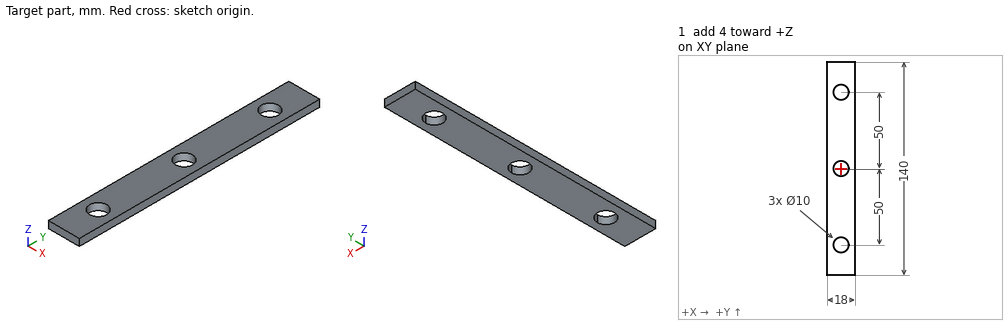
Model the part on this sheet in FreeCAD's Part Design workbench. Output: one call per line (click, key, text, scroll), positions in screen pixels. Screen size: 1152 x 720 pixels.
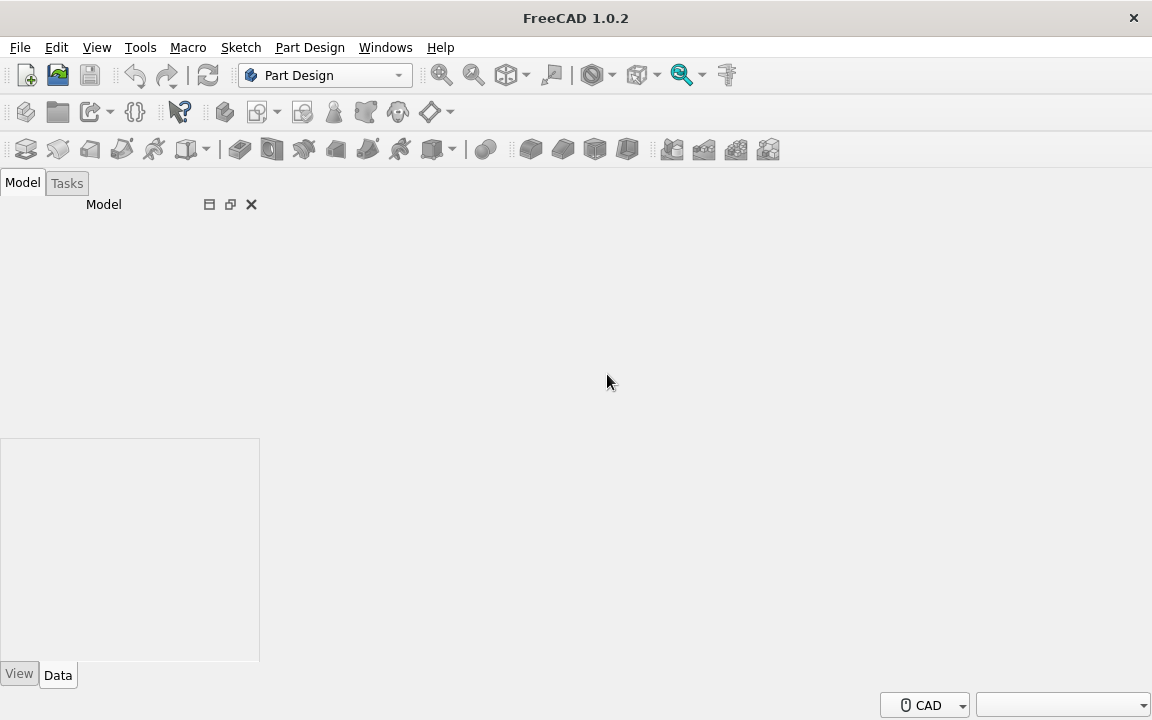
key(ctrl+n)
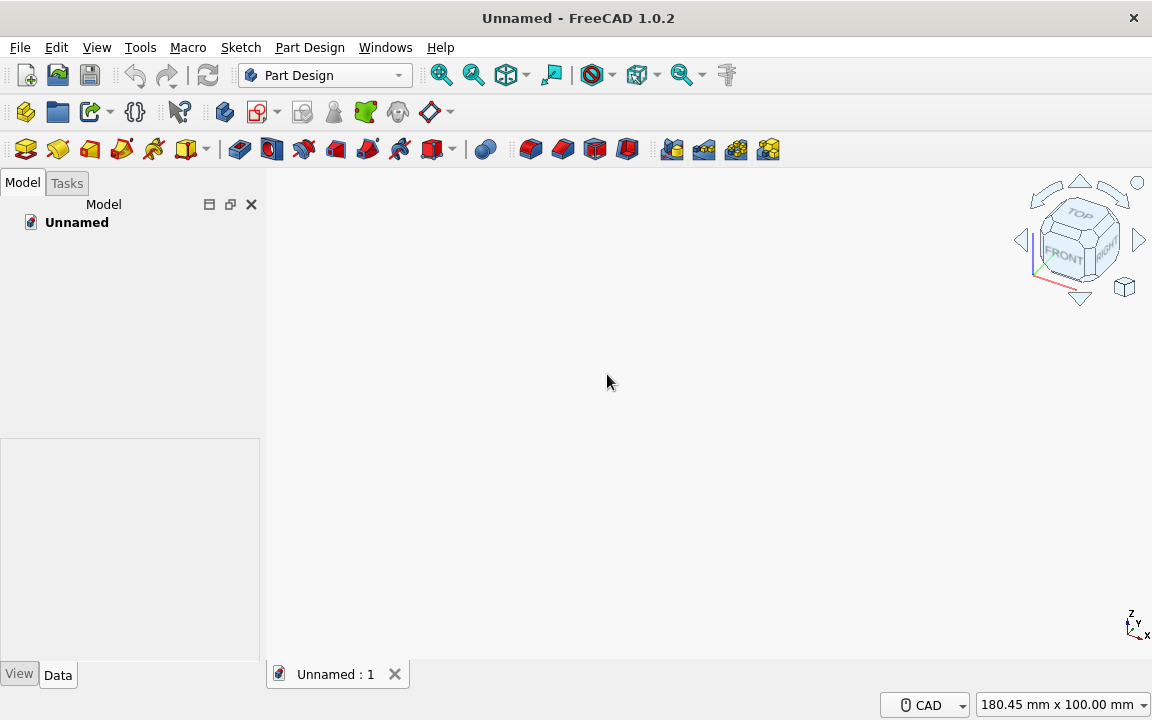
click(258, 112)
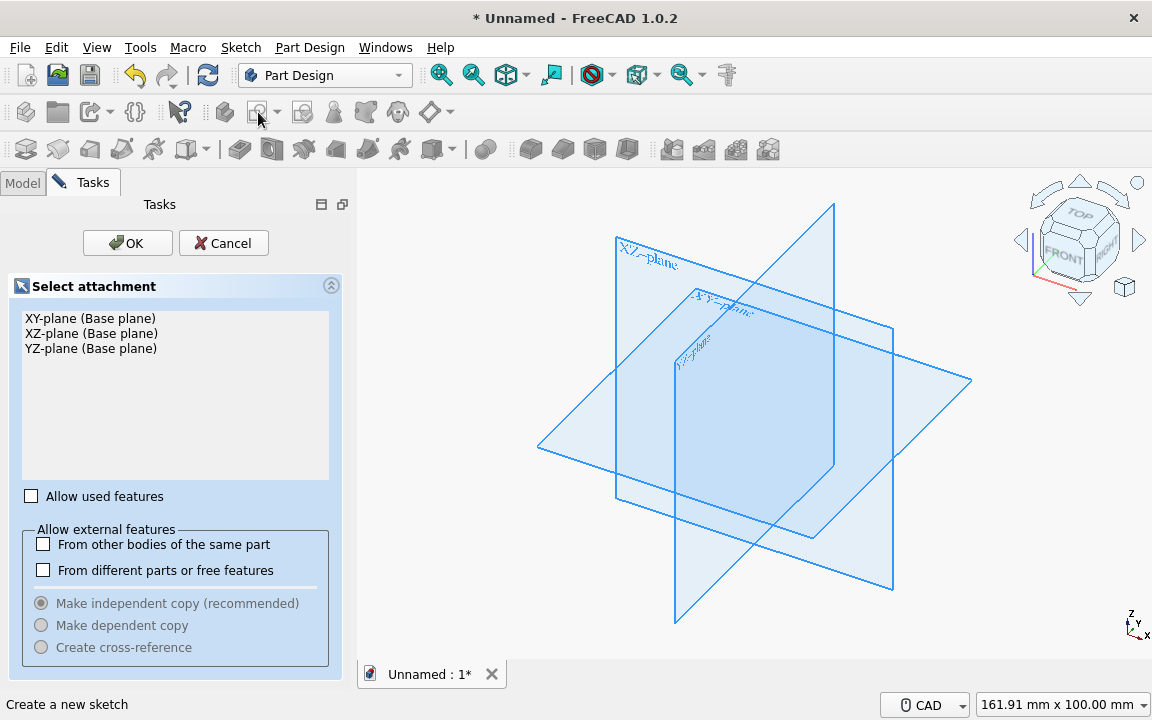
click(82, 318)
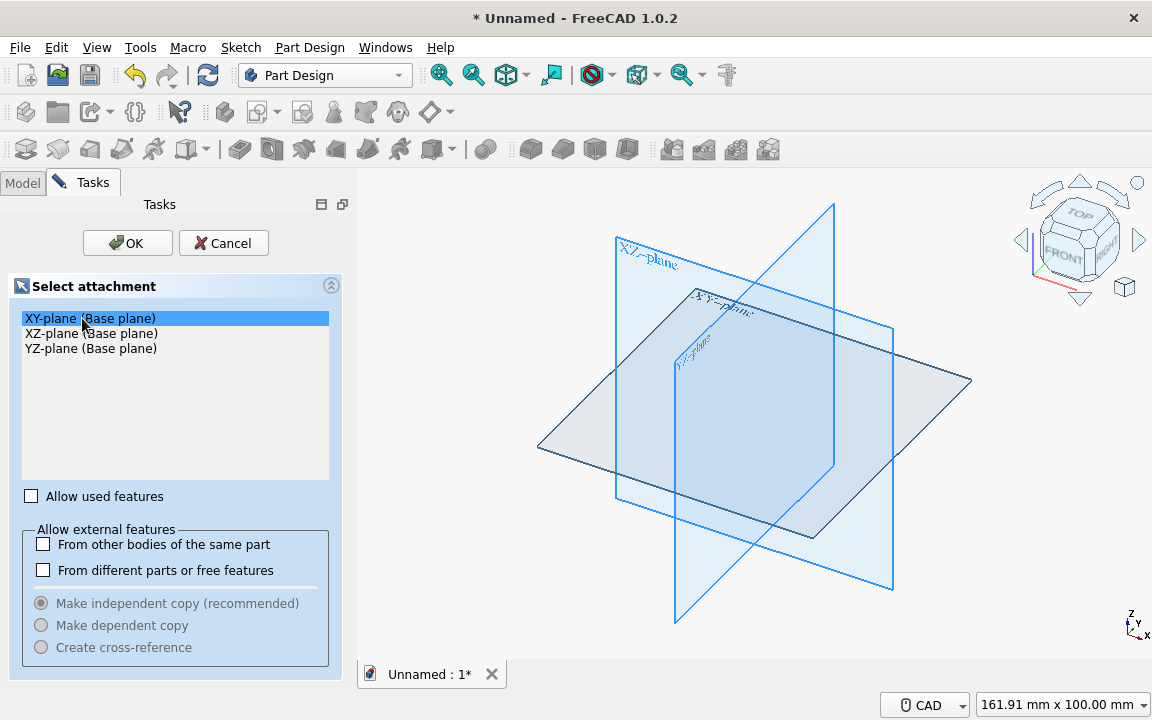
click(128, 243)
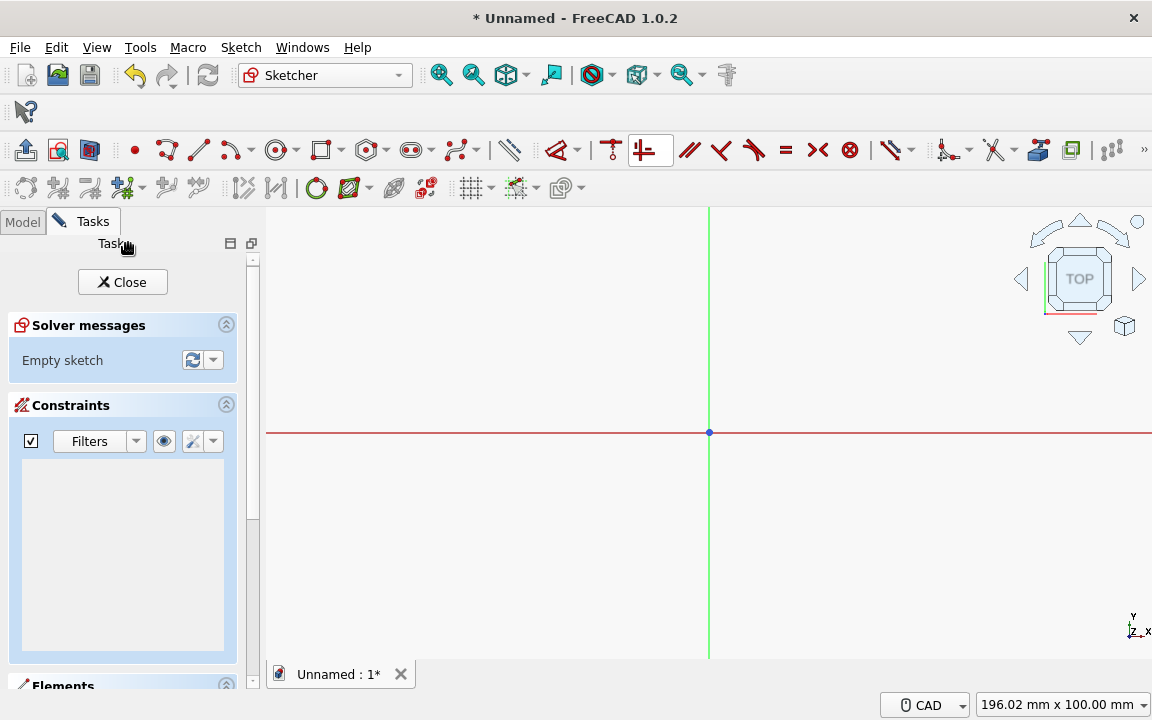
scroll(585, 433, down, 4)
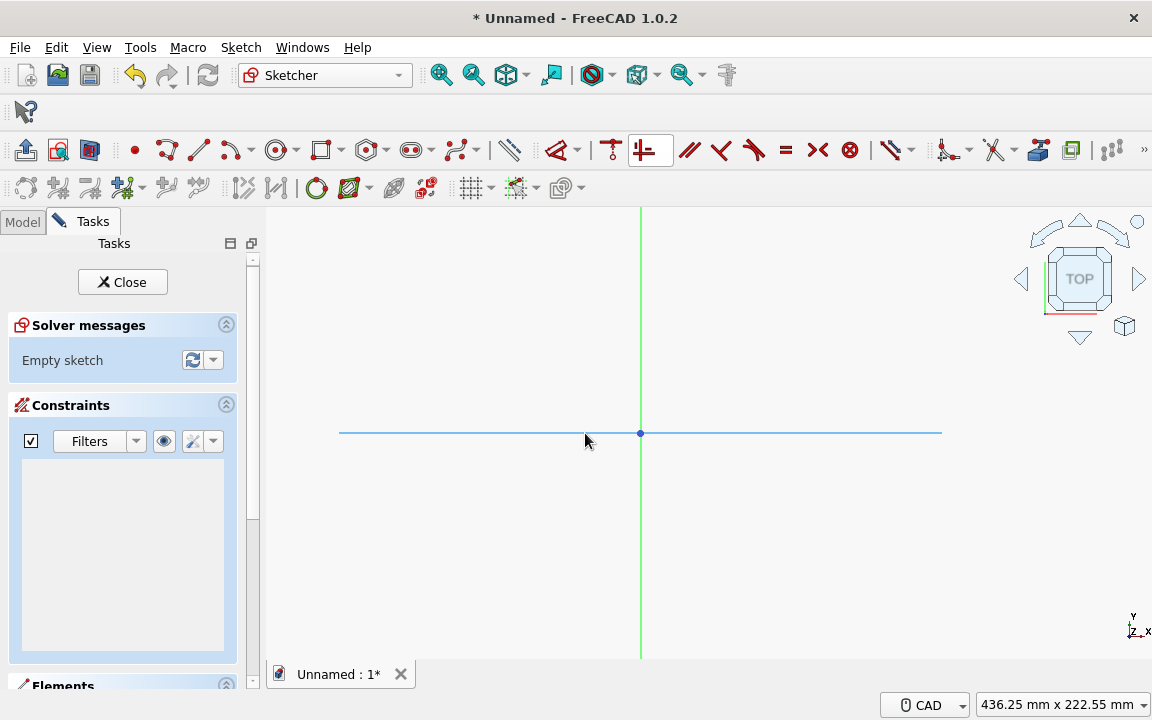
click(344, 150)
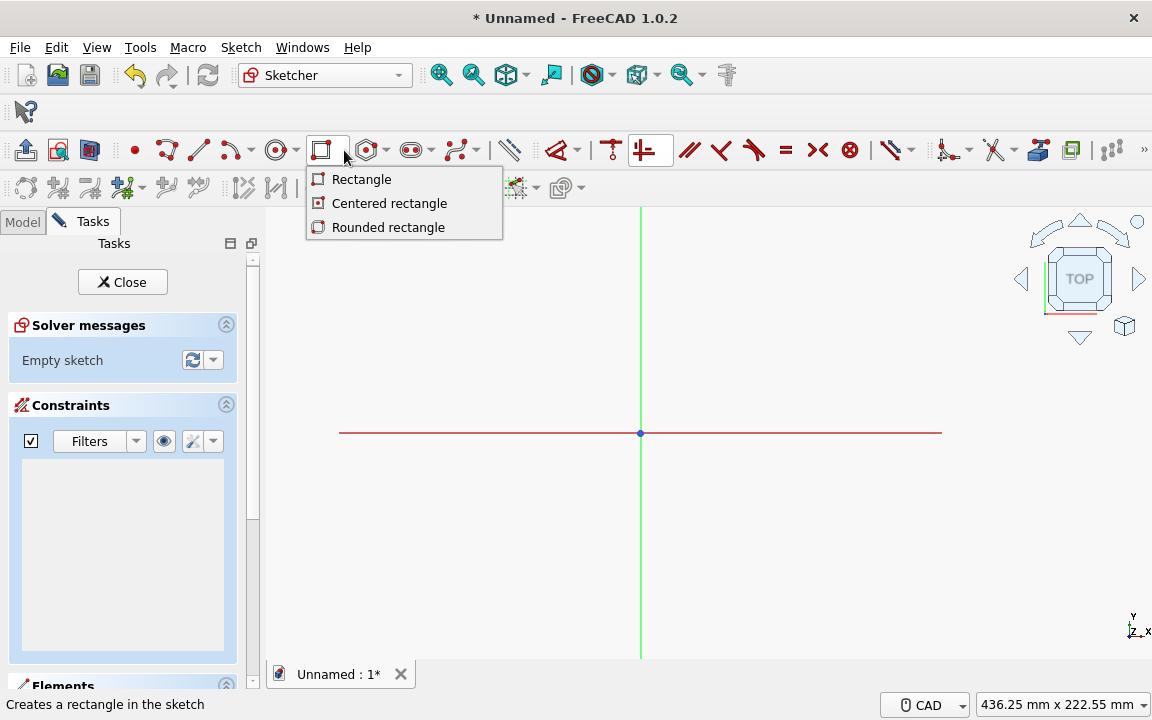
click(404, 203)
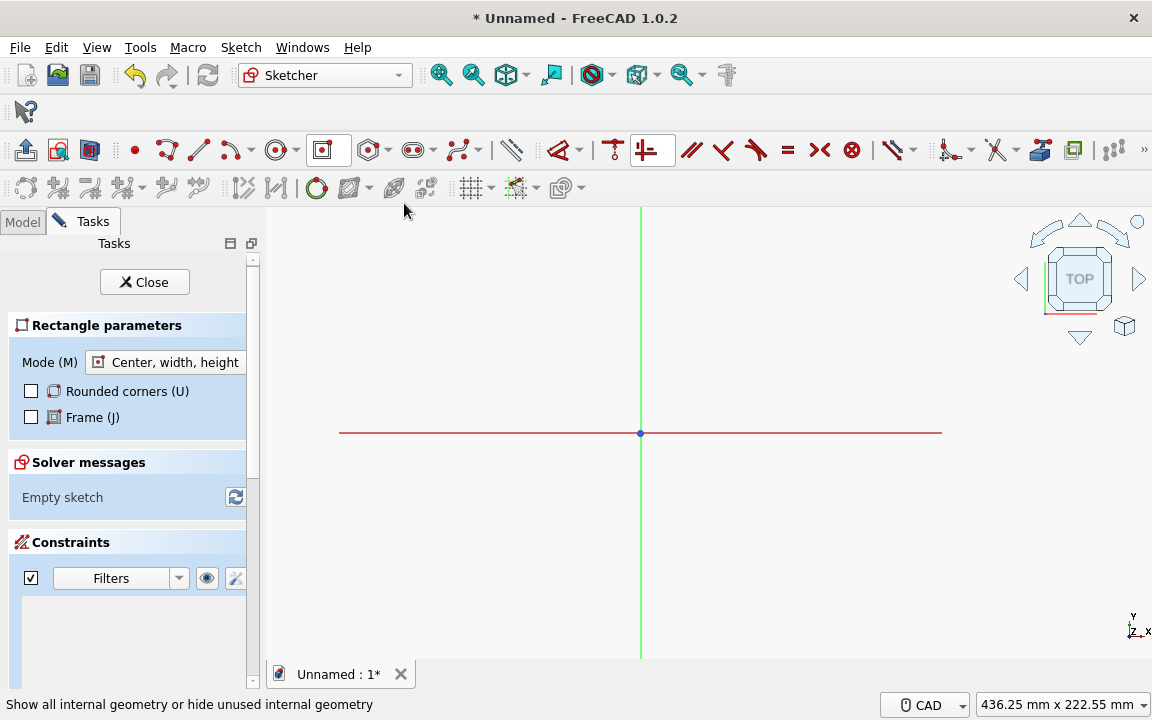
click(641, 433)
move(659, 291)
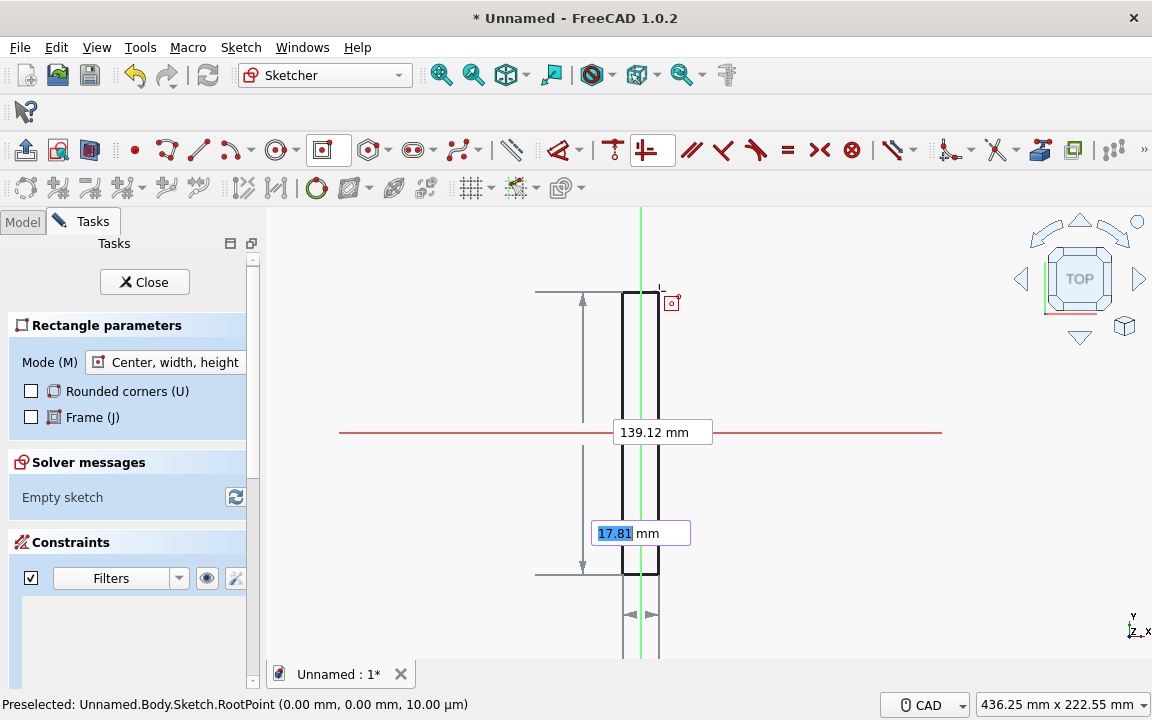
text(18)
key(Tab)
text(140)
key(Return)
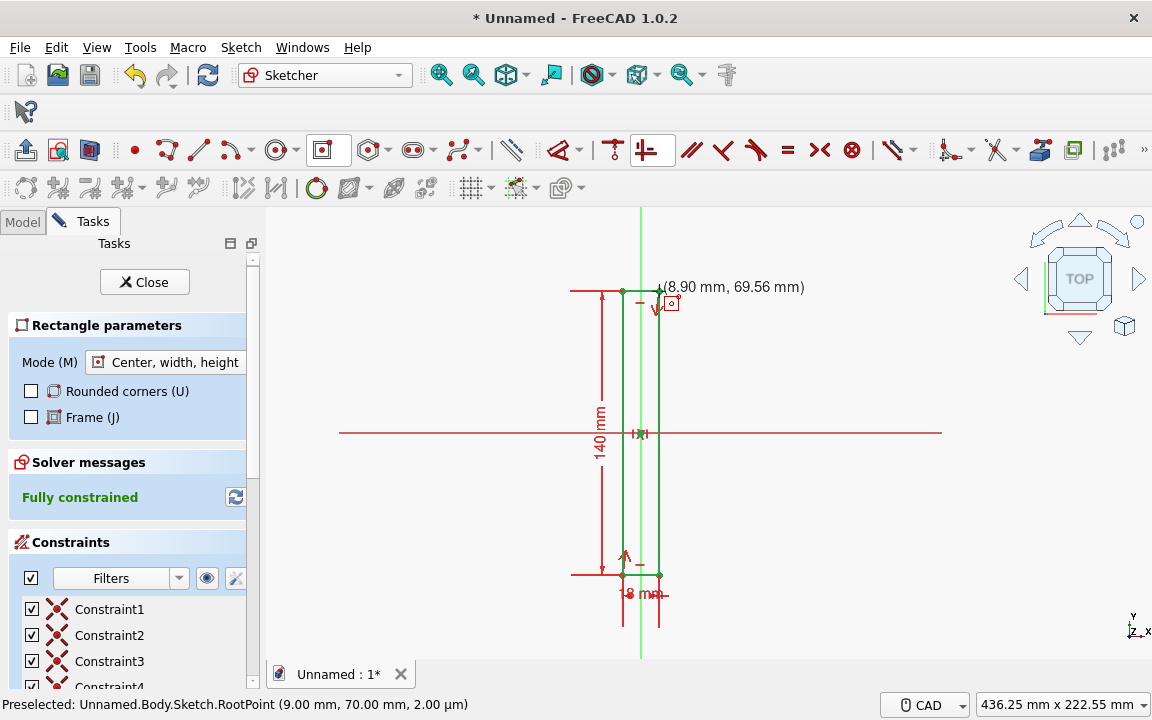
key(g)
key(c)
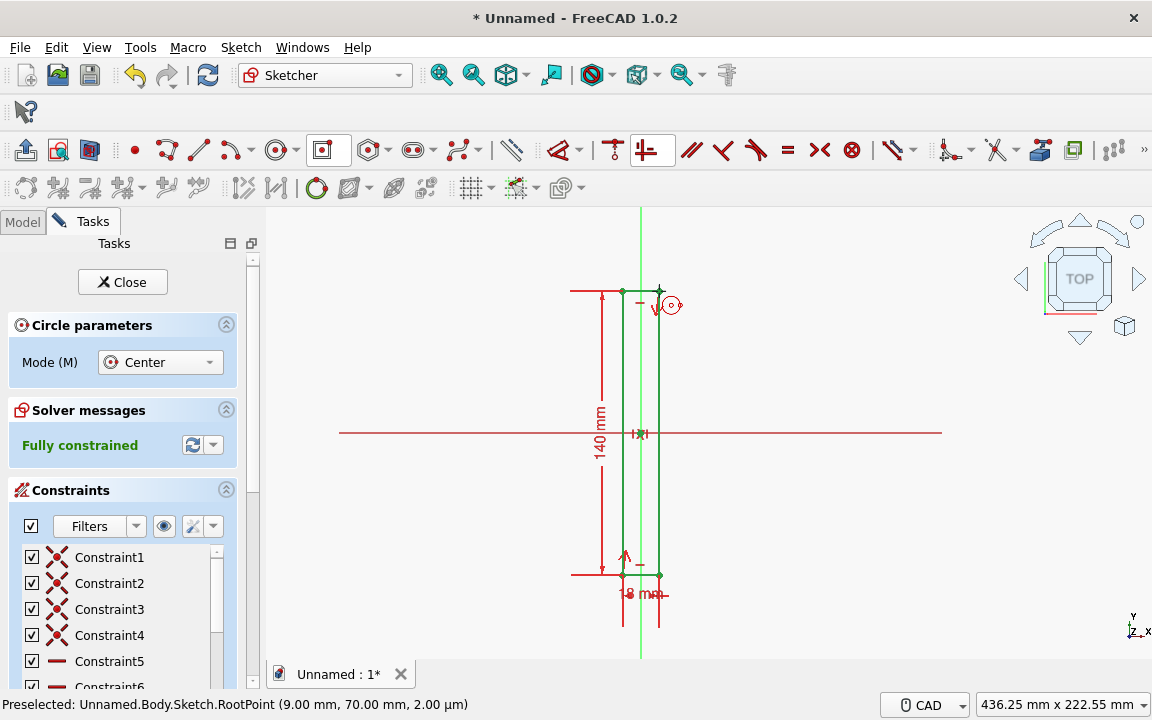
scroll(641, 535, up, 5)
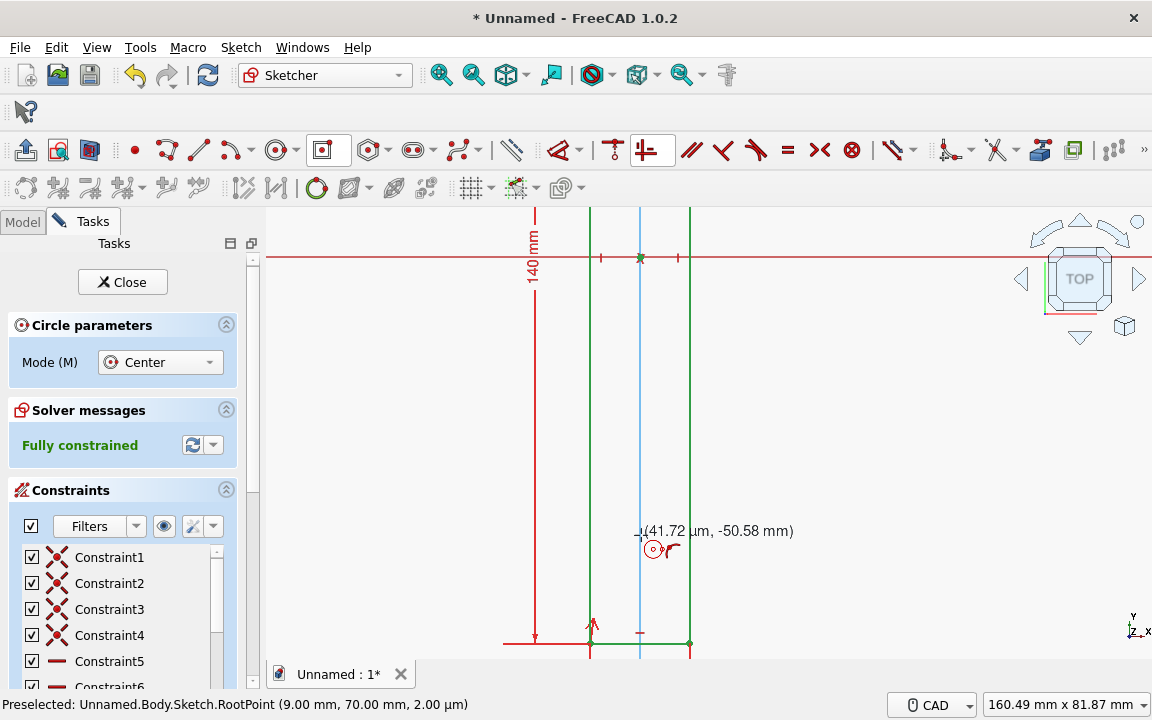
click(640, 533)
move(660, 514)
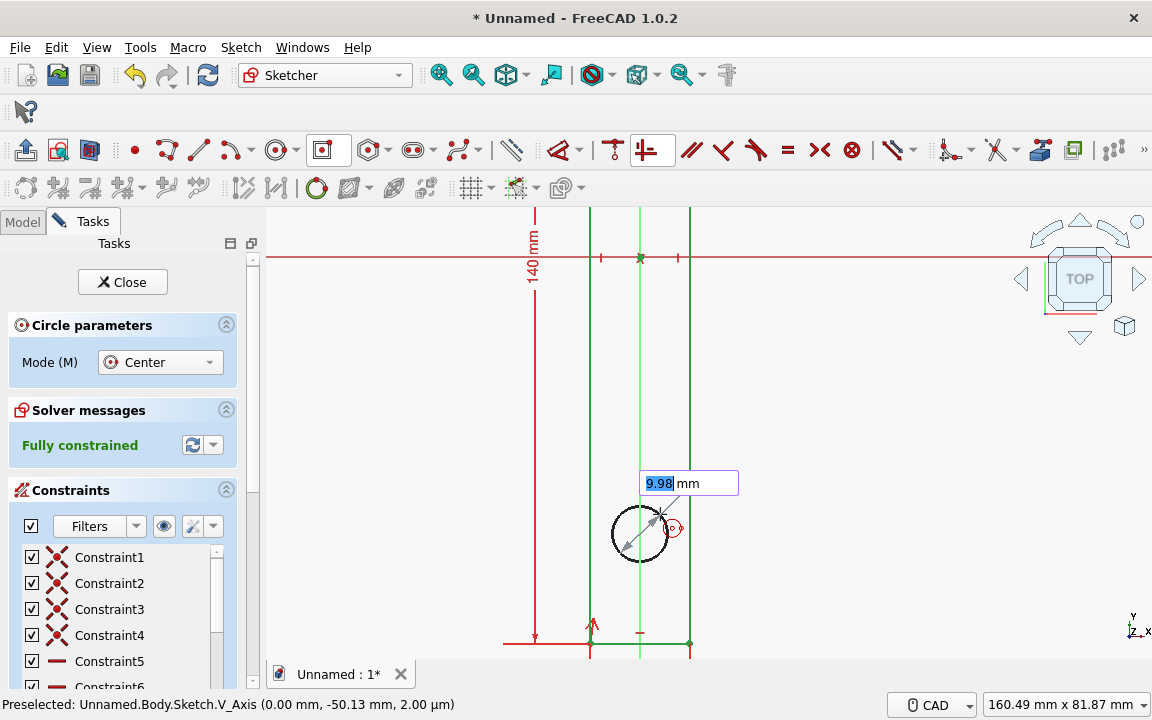
text(10)
key(Return)